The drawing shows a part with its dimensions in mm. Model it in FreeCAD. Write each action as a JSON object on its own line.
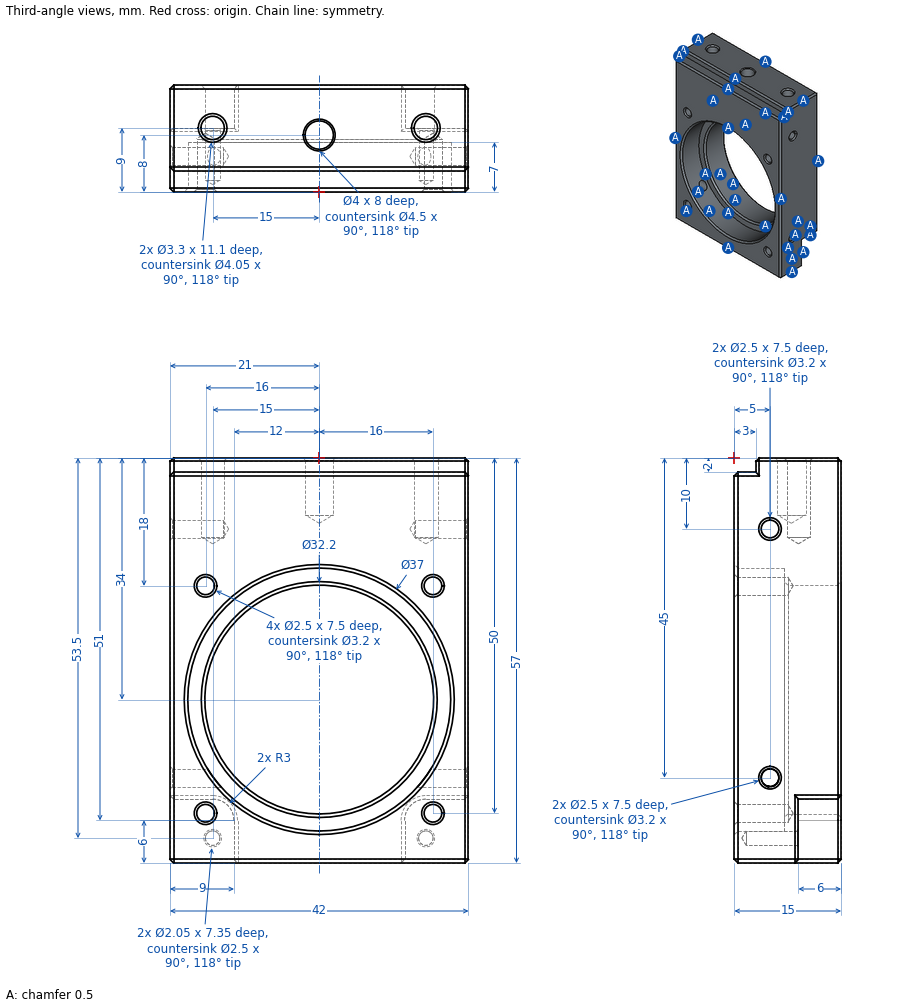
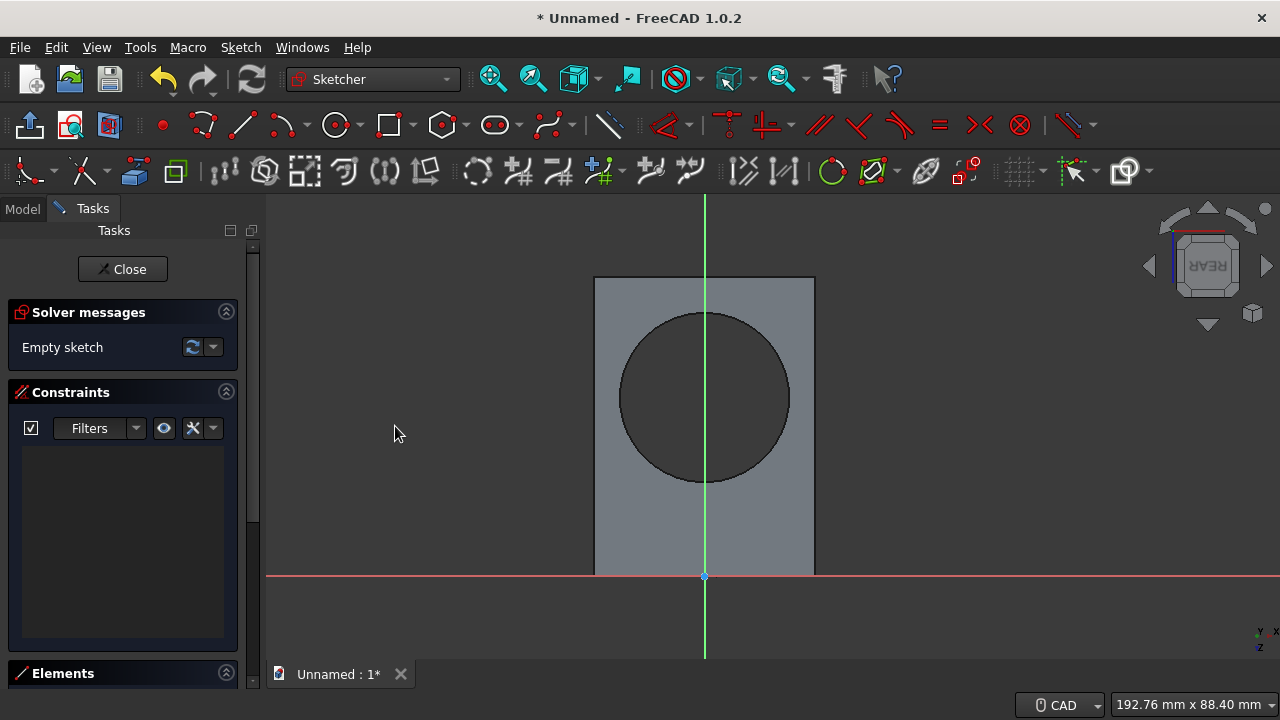
{"action": "key", "text": "g m"}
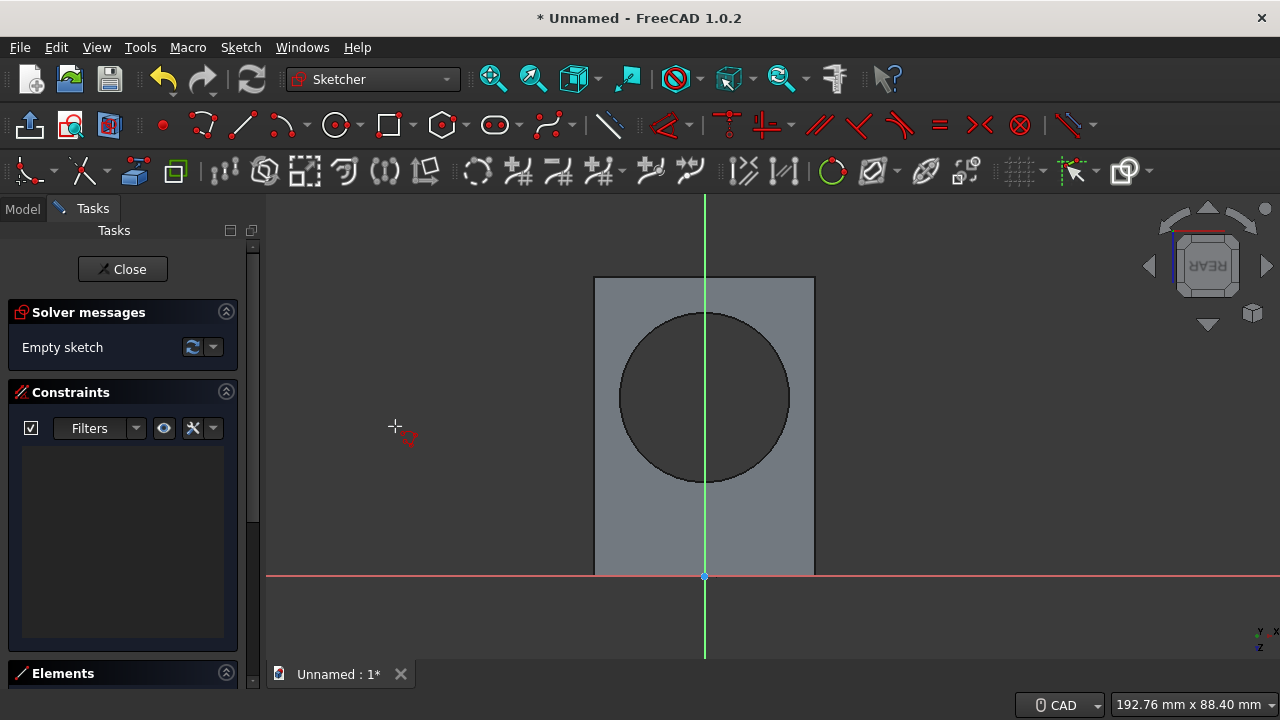
{"action": "left_click", "coordinate": [641, 308]}
{"action": "left_click", "coordinate": [641, 277]}
{"action": "left_click", "coordinate": [594, 277]}
{"action": "left_click", "coordinate": [594, 324]}
{"action": "left_click", "coordinate": [626, 324]}
{"action": "right_click", "coordinate": [626, 324]}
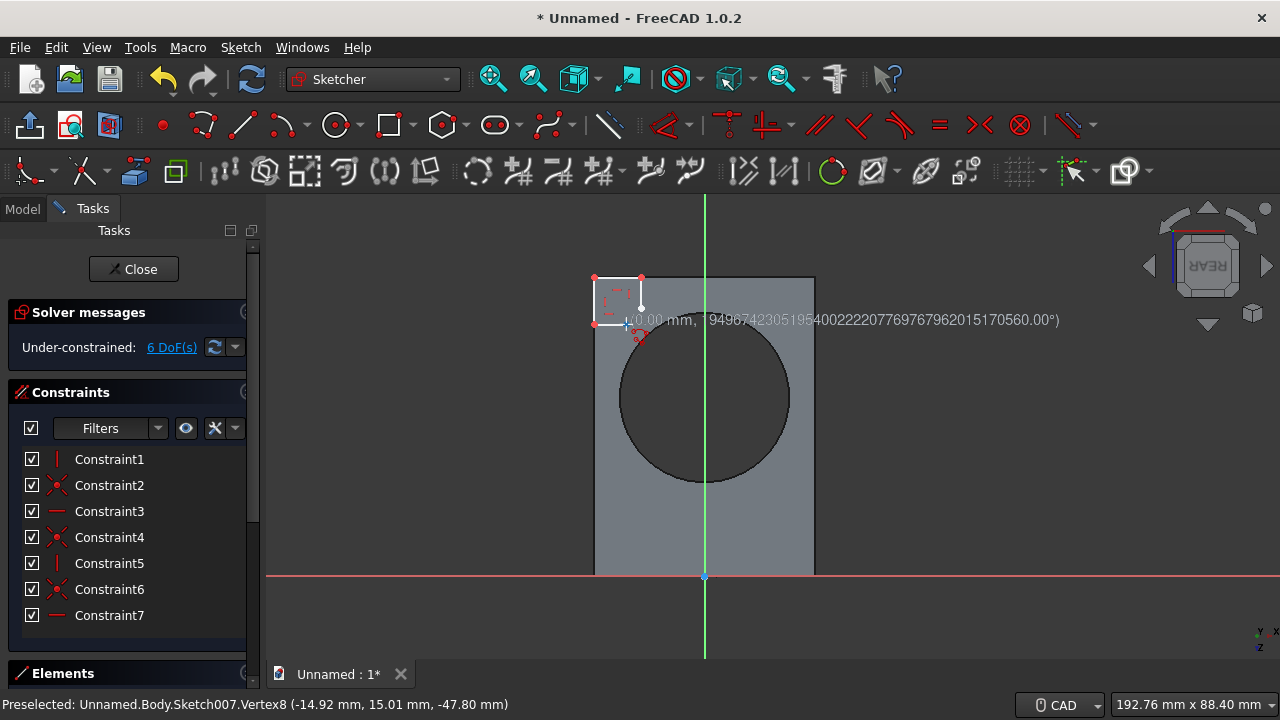
{"action": "left_click", "coordinate": [310, 126]}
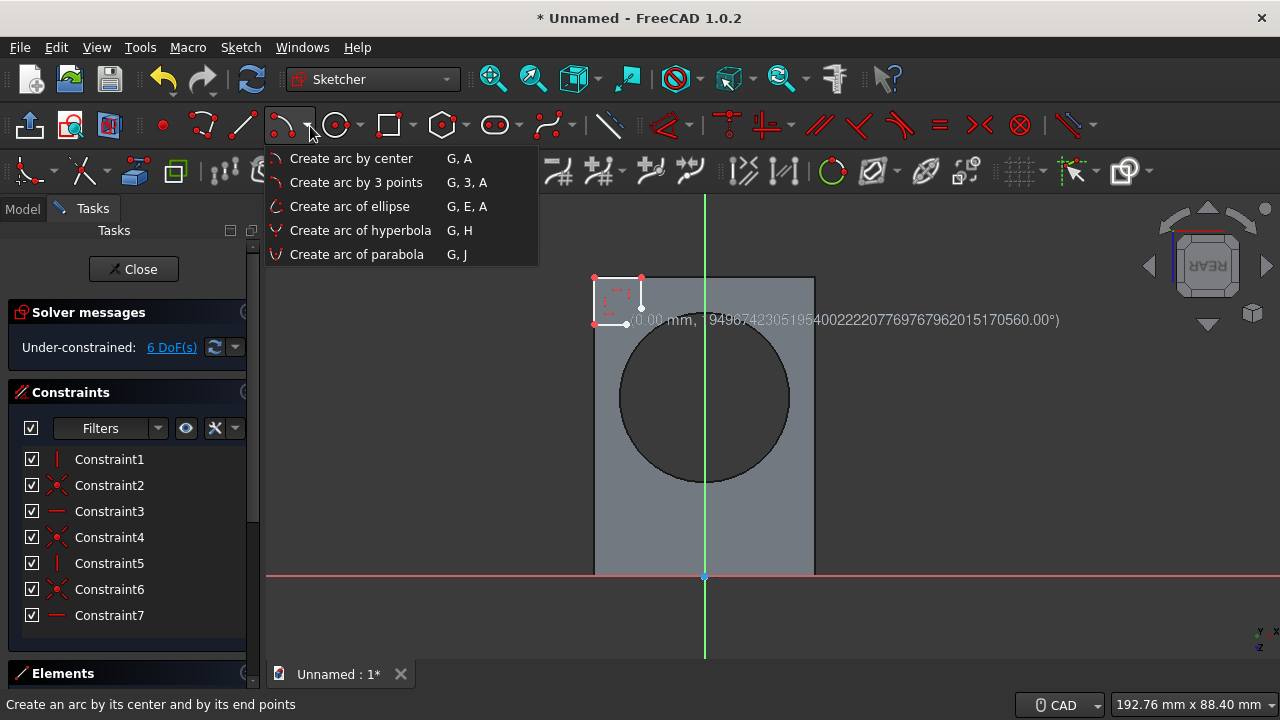
{"action": "left_click", "coordinate": [402, 182]}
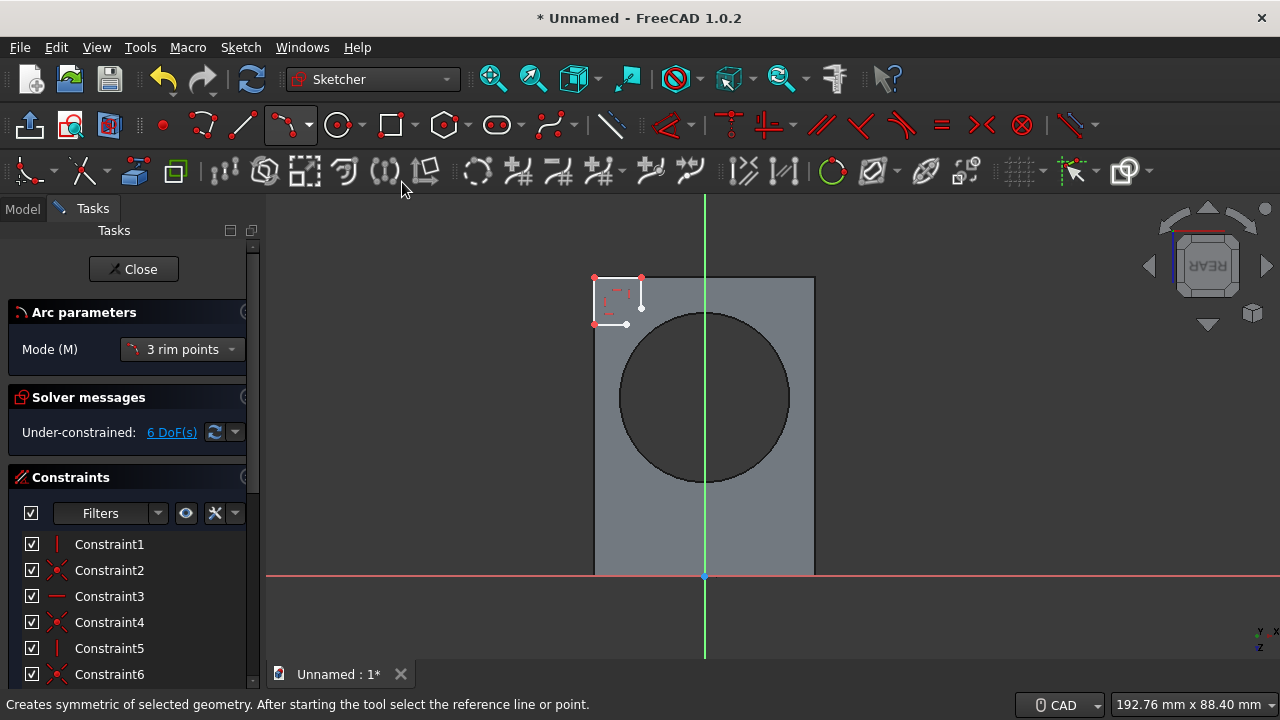
{"action": "left_click", "coordinate": [626, 325]}
{"action": "left_click", "coordinate": [641, 309]}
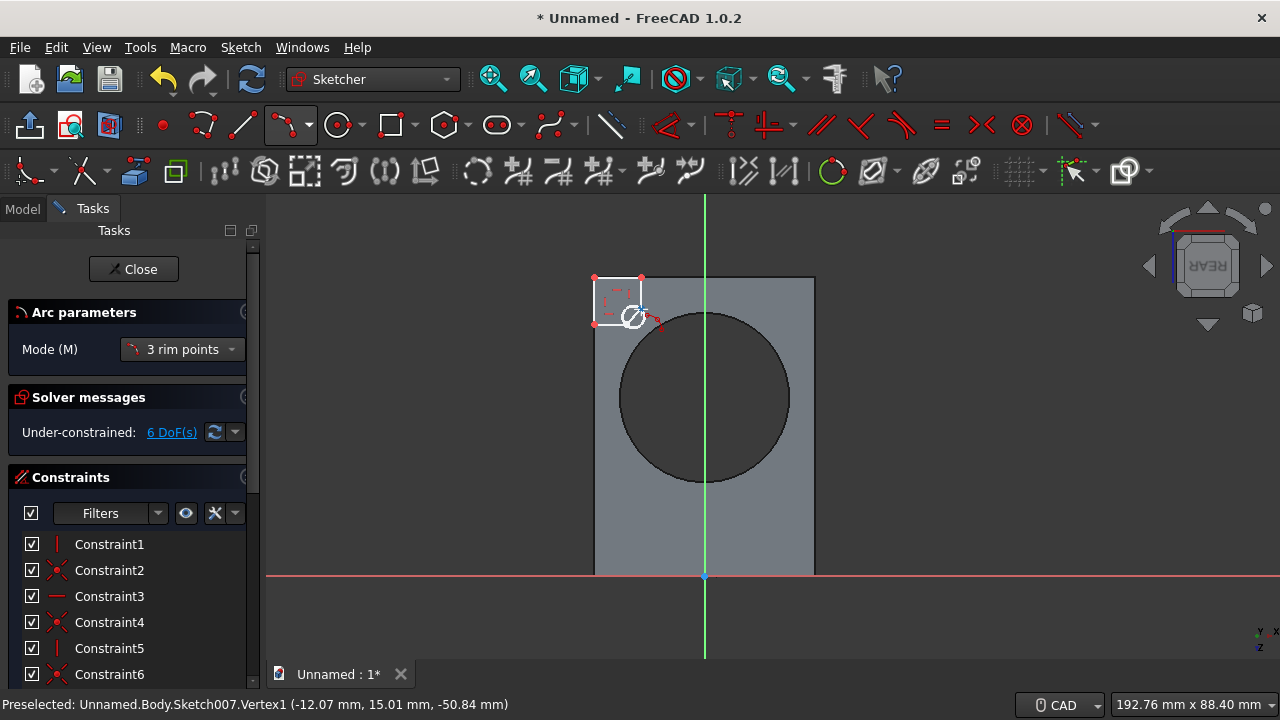
{"action": "scroll", "coordinate": [637, 319], "scroll_direction": "up", "scroll_amount": 7}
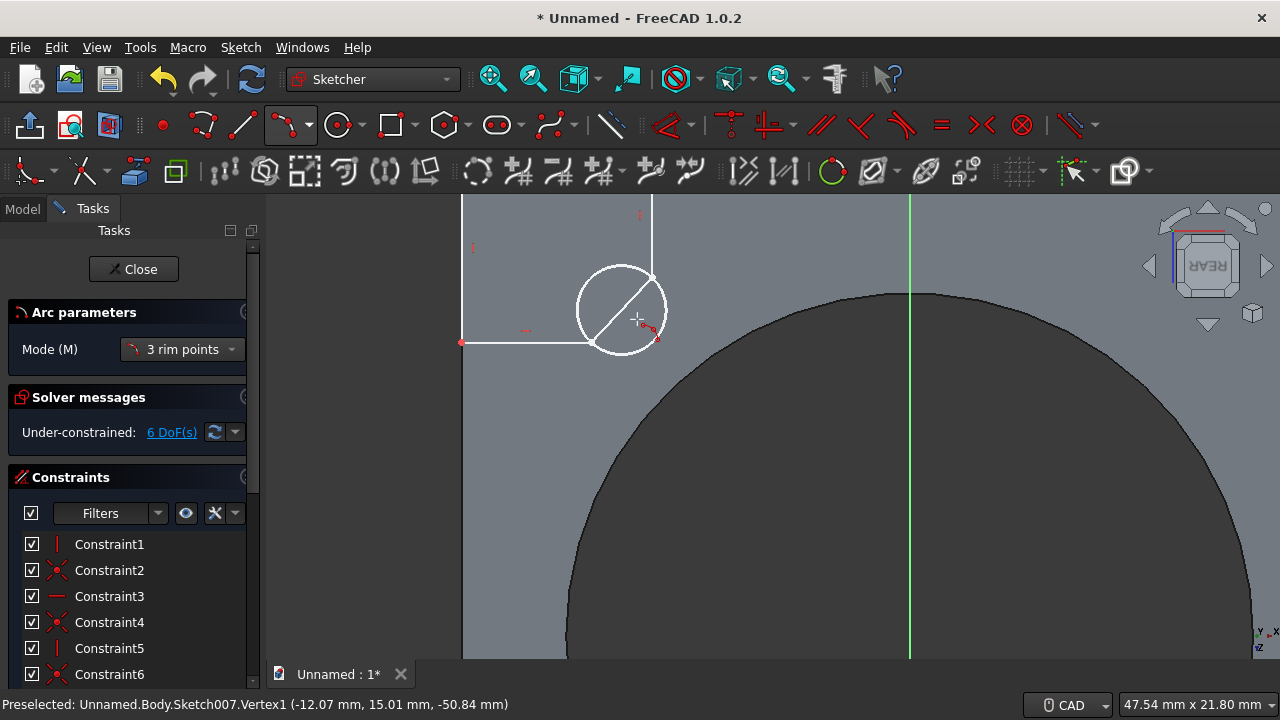
{"action": "left_click", "coordinate": [635, 319]}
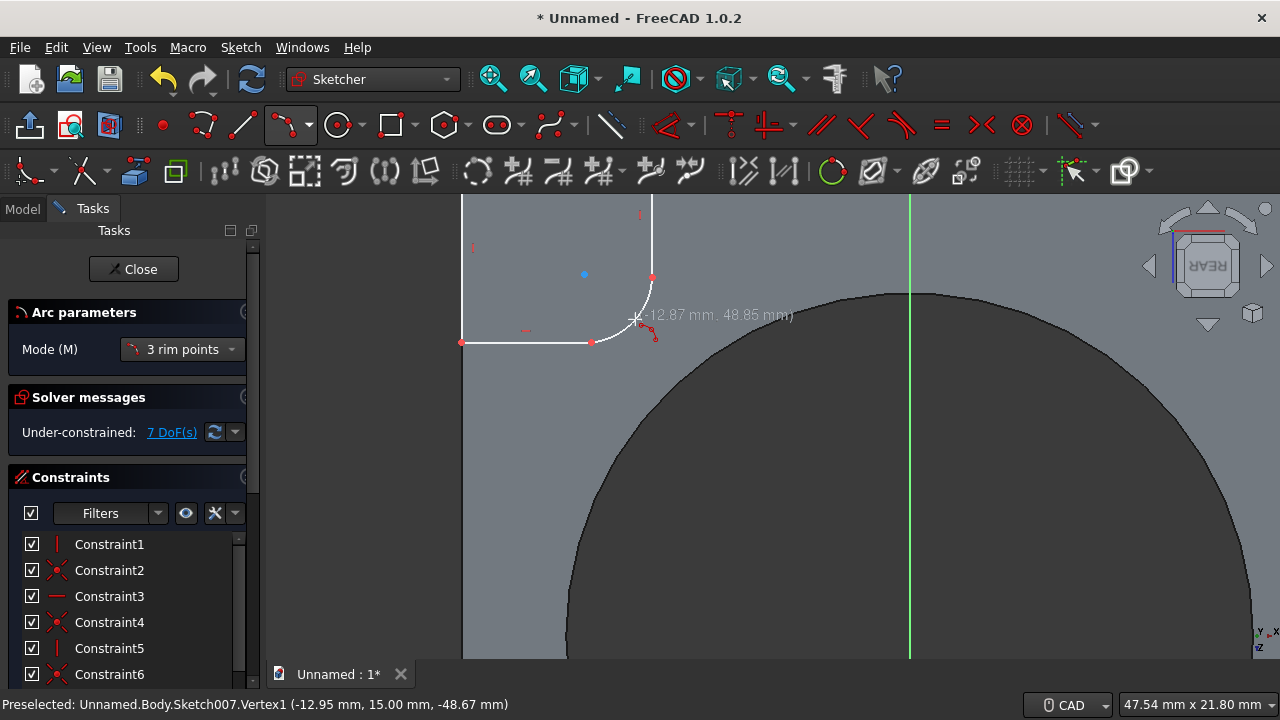
{"action": "left_click", "coordinate": [204, 126]}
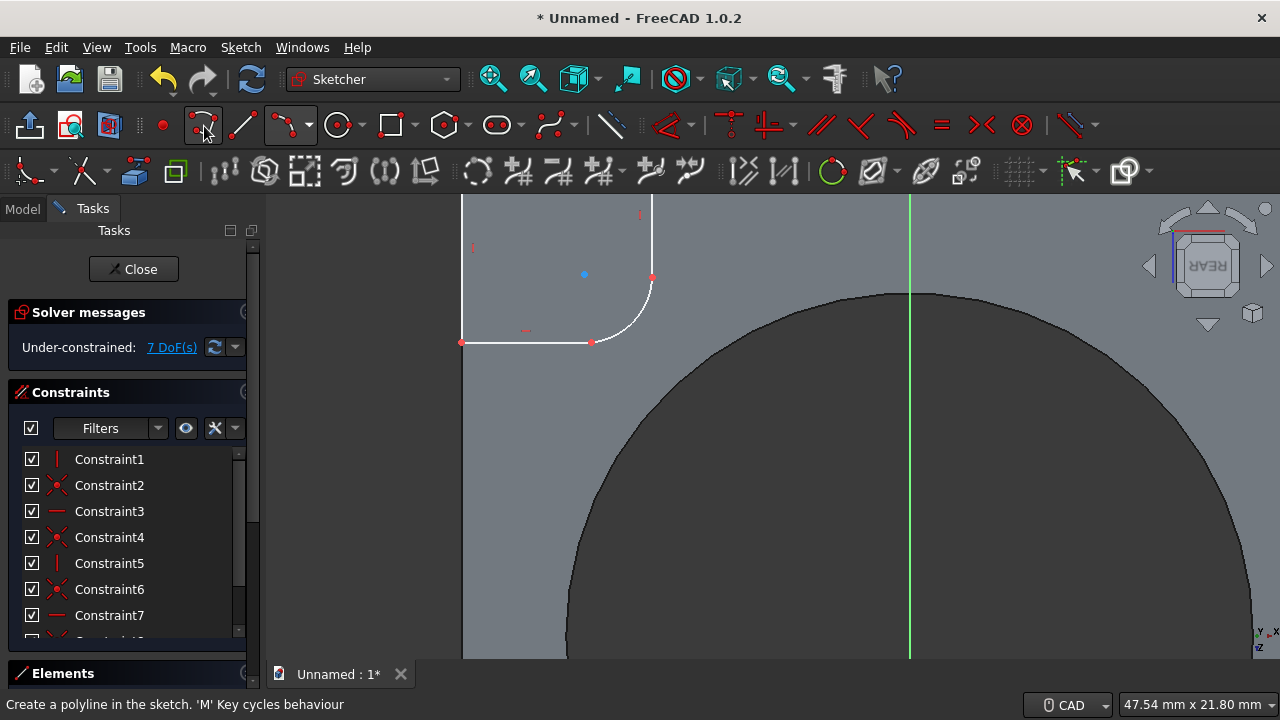
{"action": "scroll", "coordinate": [637, 319], "scroll_direction": "down", "scroll_amount": 7}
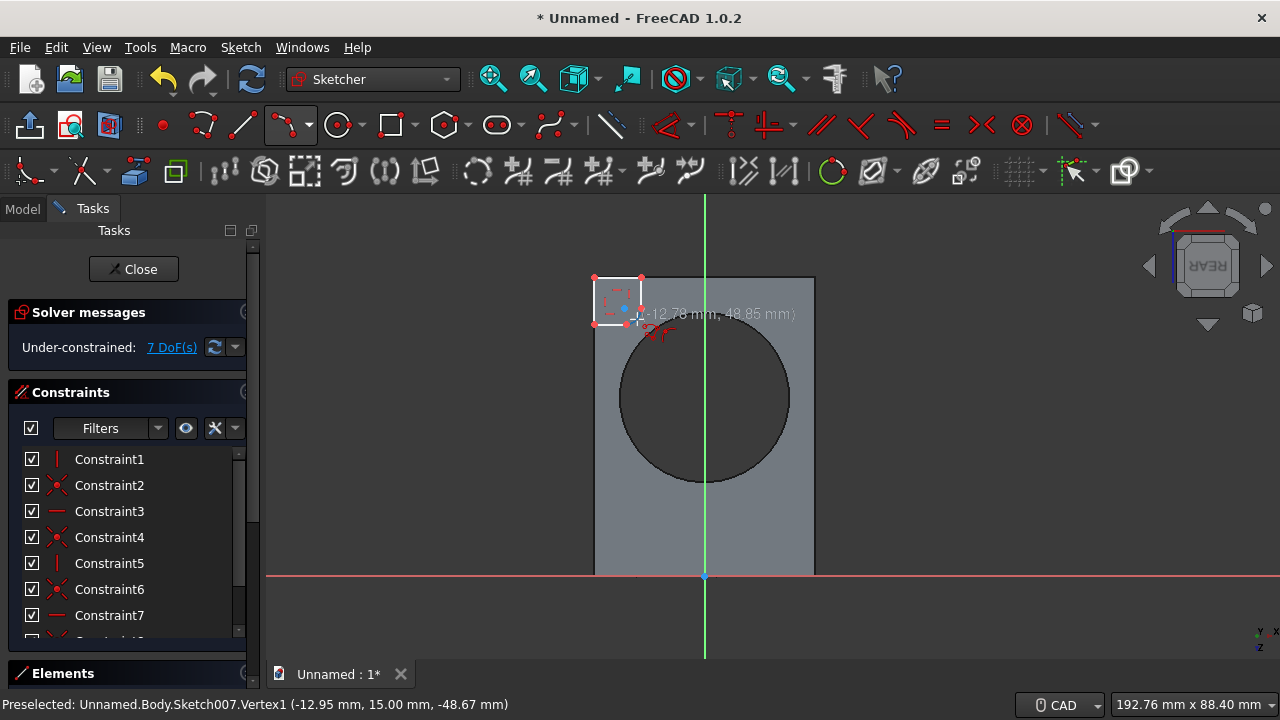
{"action": "left_click", "coordinate": [783, 324]}
{"action": "left_click", "coordinate": [815, 324]}
{"action": "left_click", "coordinate": [815, 277]}
{"action": "left_click", "coordinate": [768, 277]}
{"action": "left_click", "coordinate": [768, 308]}
{"action": "right_click", "coordinate": [768, 308]}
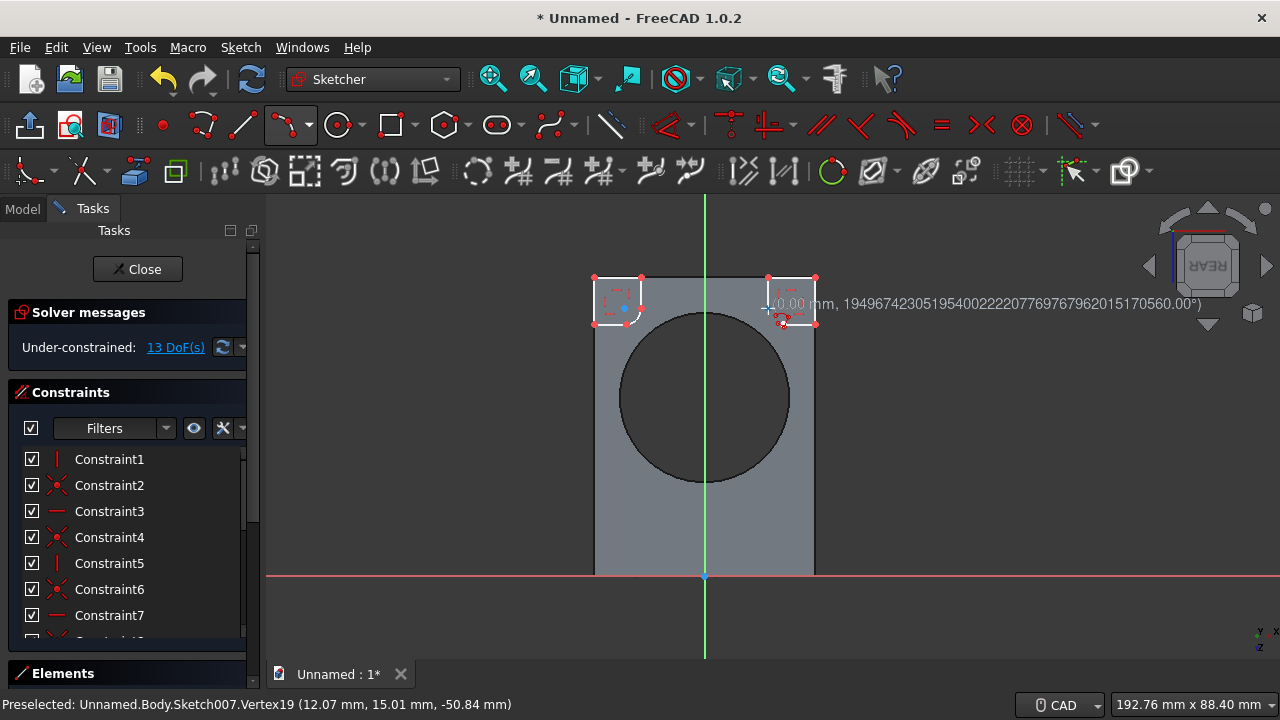
{"action": "left_click", "coordinate": [284, 126]}